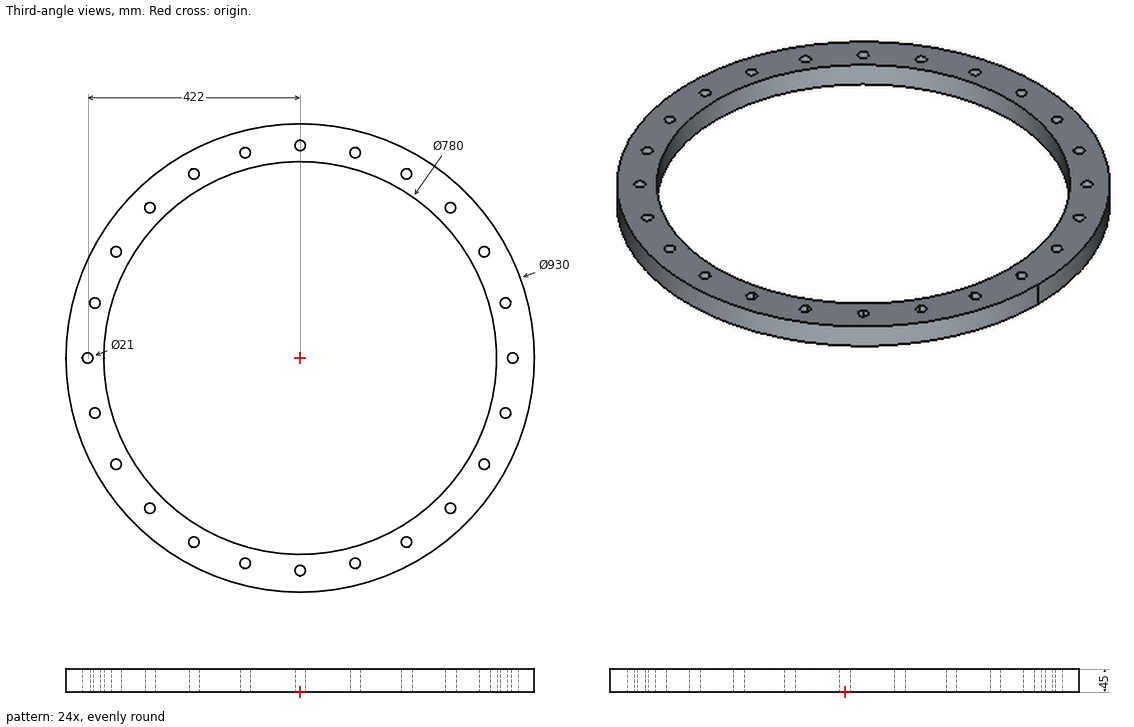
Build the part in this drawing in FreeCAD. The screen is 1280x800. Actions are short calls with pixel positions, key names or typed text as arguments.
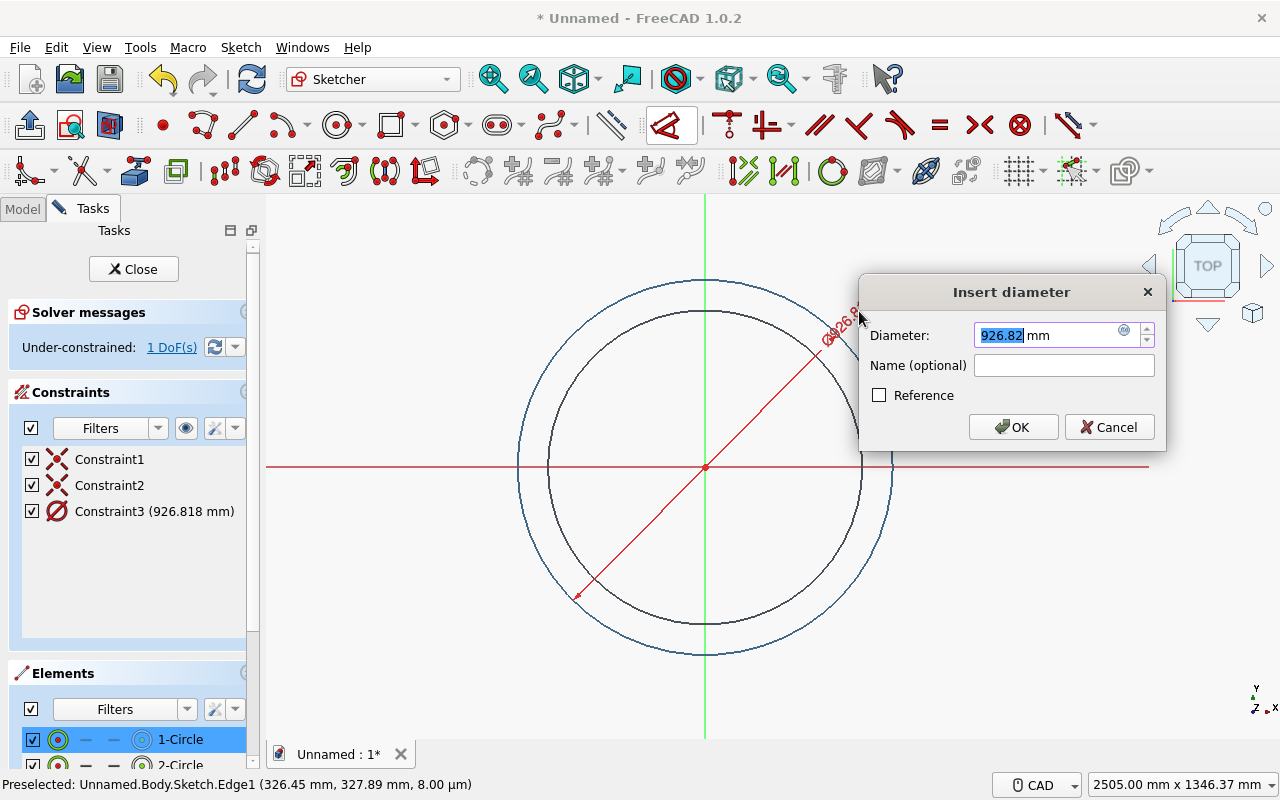
text(930)
key(Return)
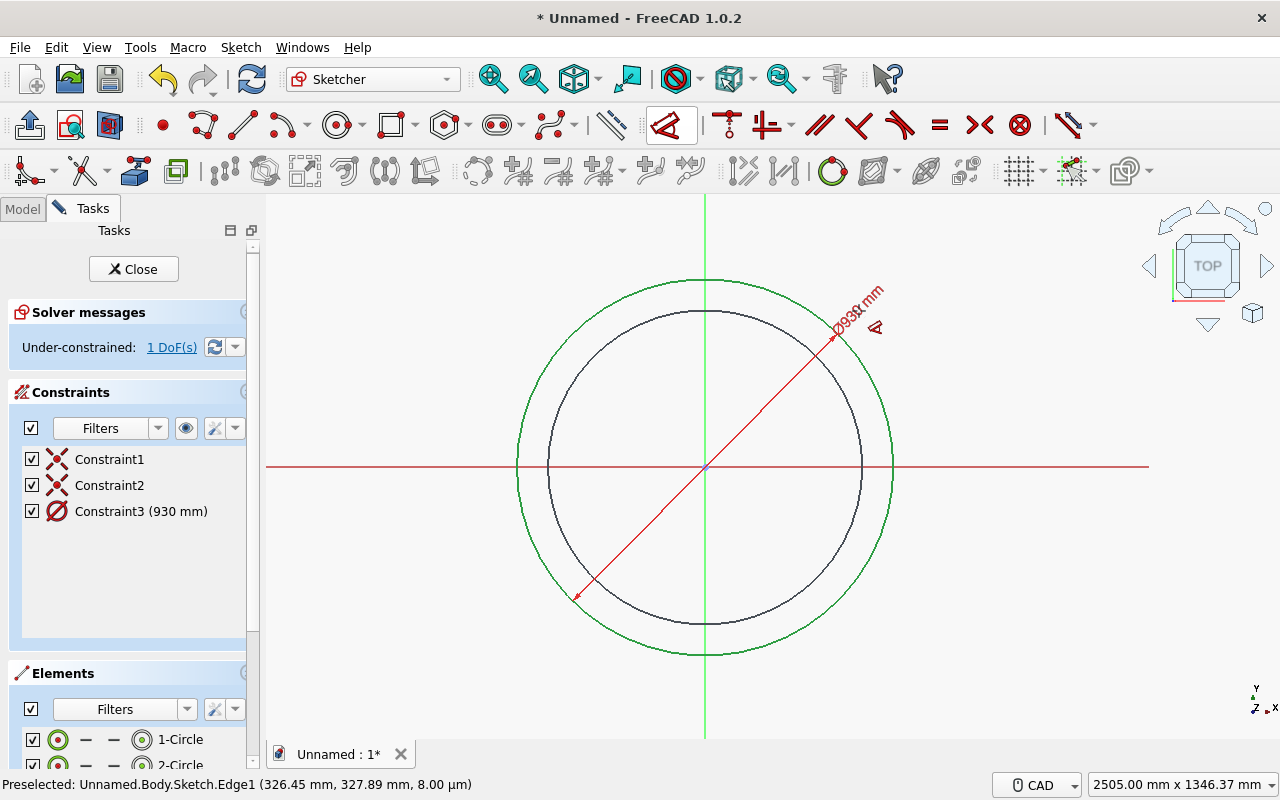
click(816, 356)
click(909, 407)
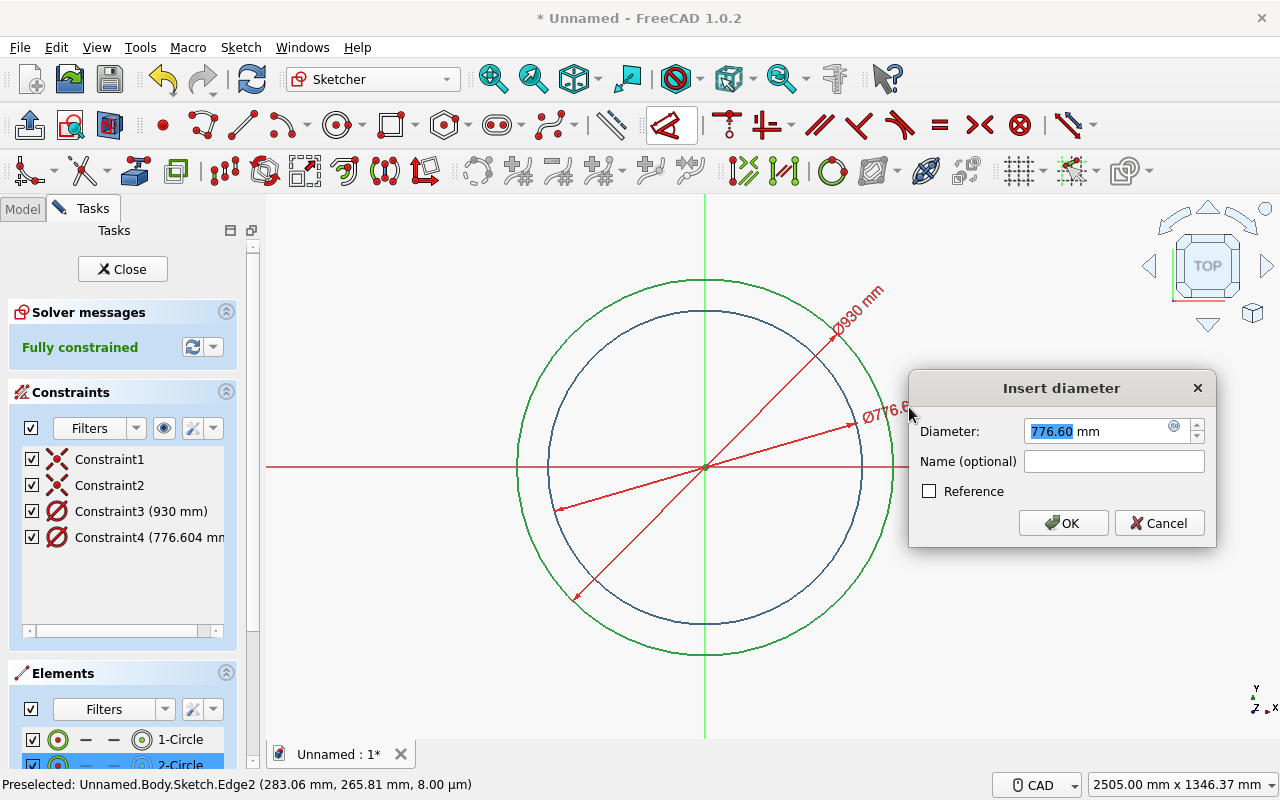
text(780)
key(Return)
key(Escape)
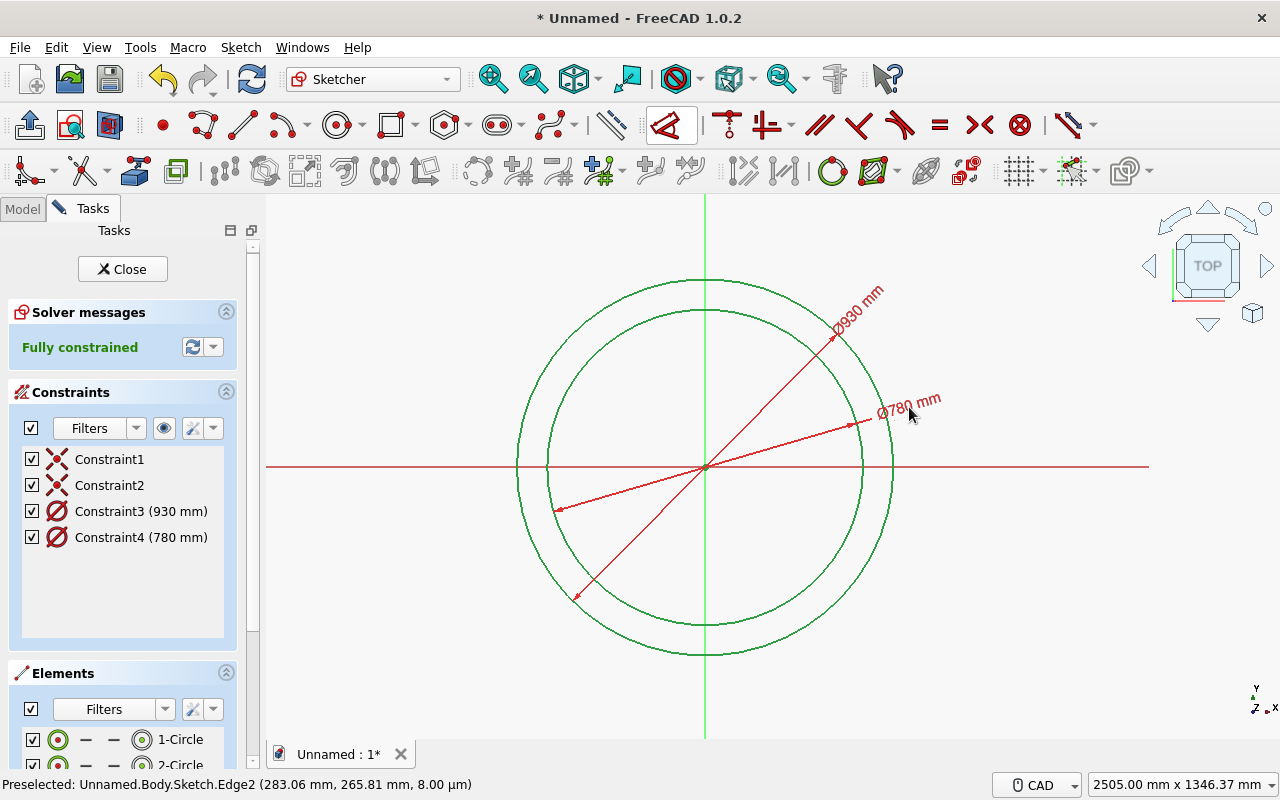
click(123, 269)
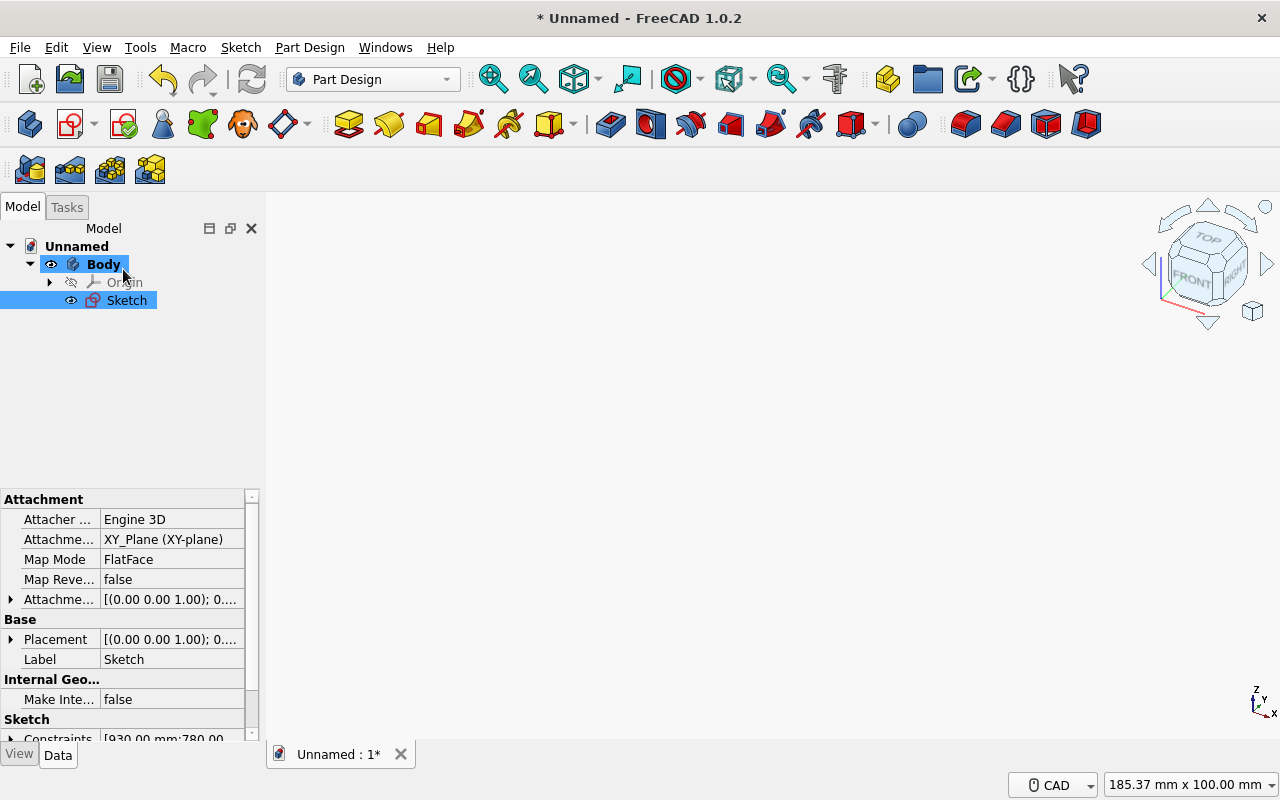
click(350, 124)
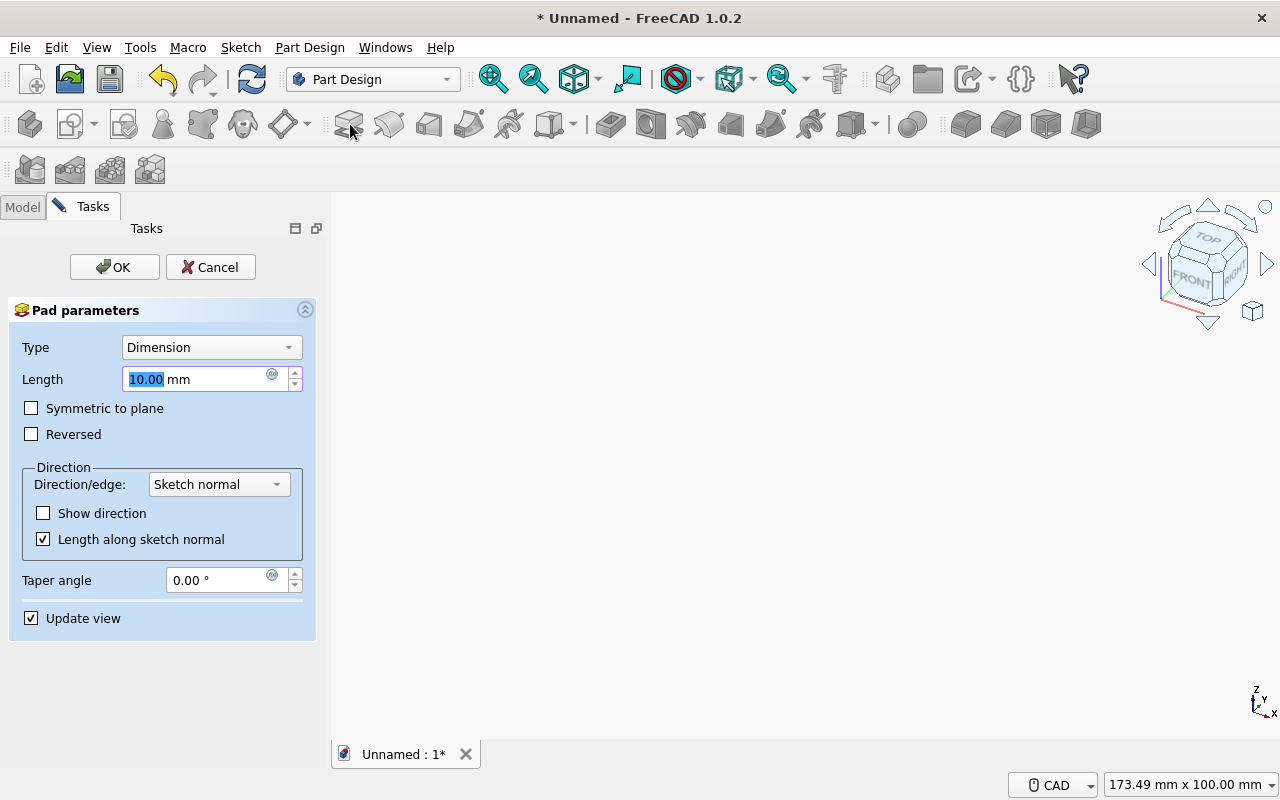
text(45)
key(Tab)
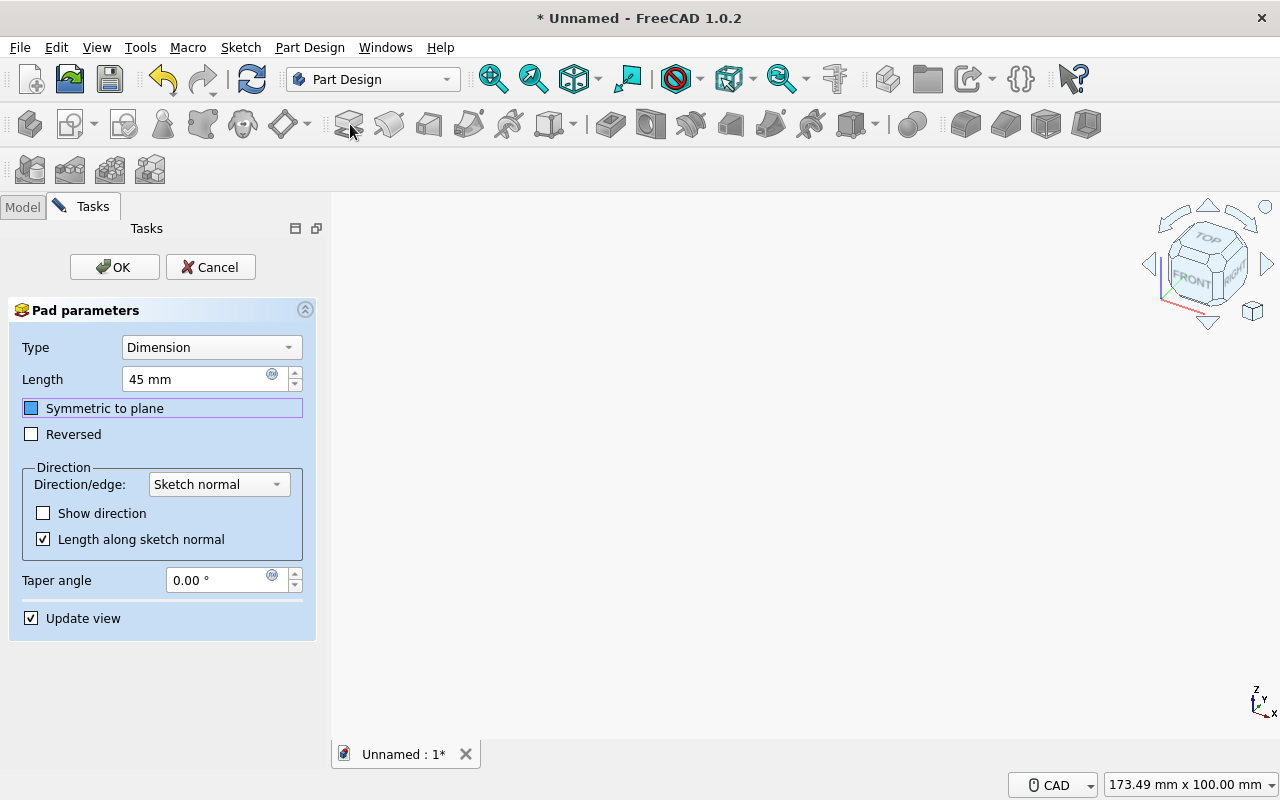
click(115, 267)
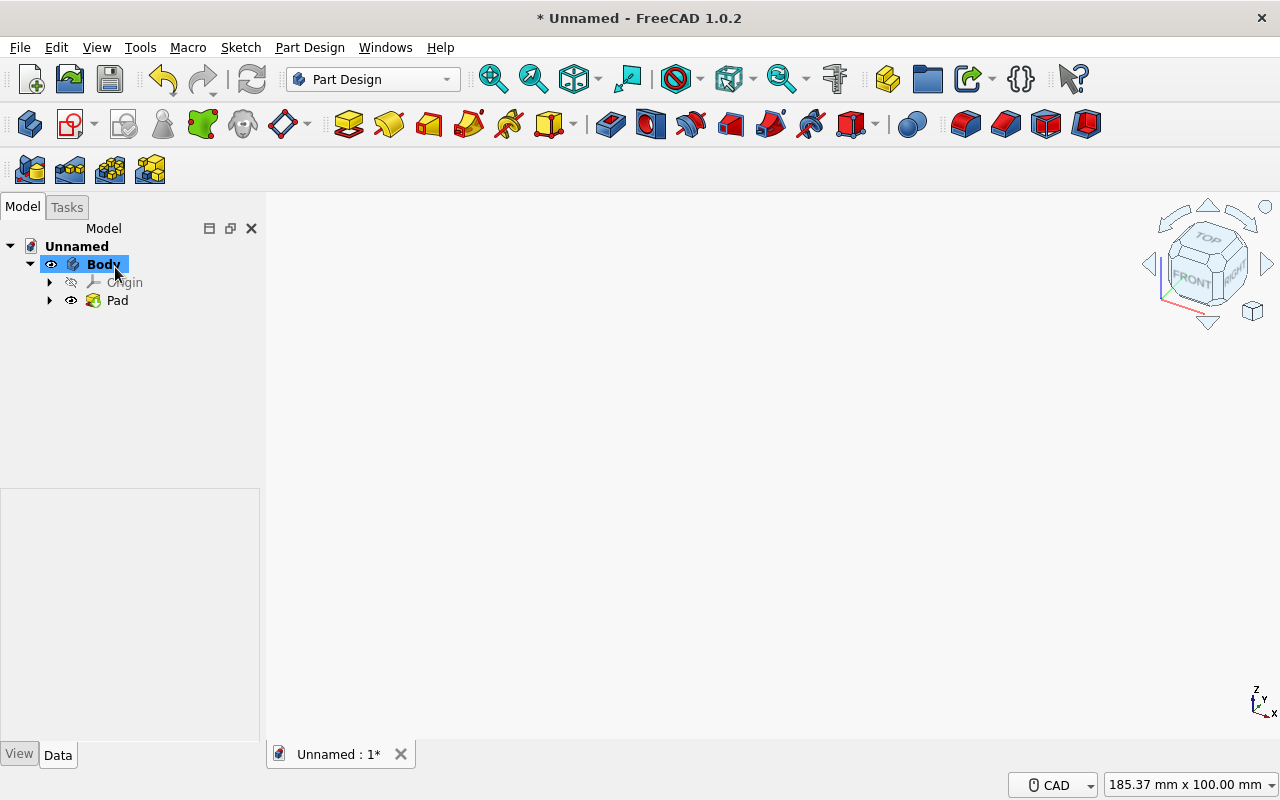
click(494, 80)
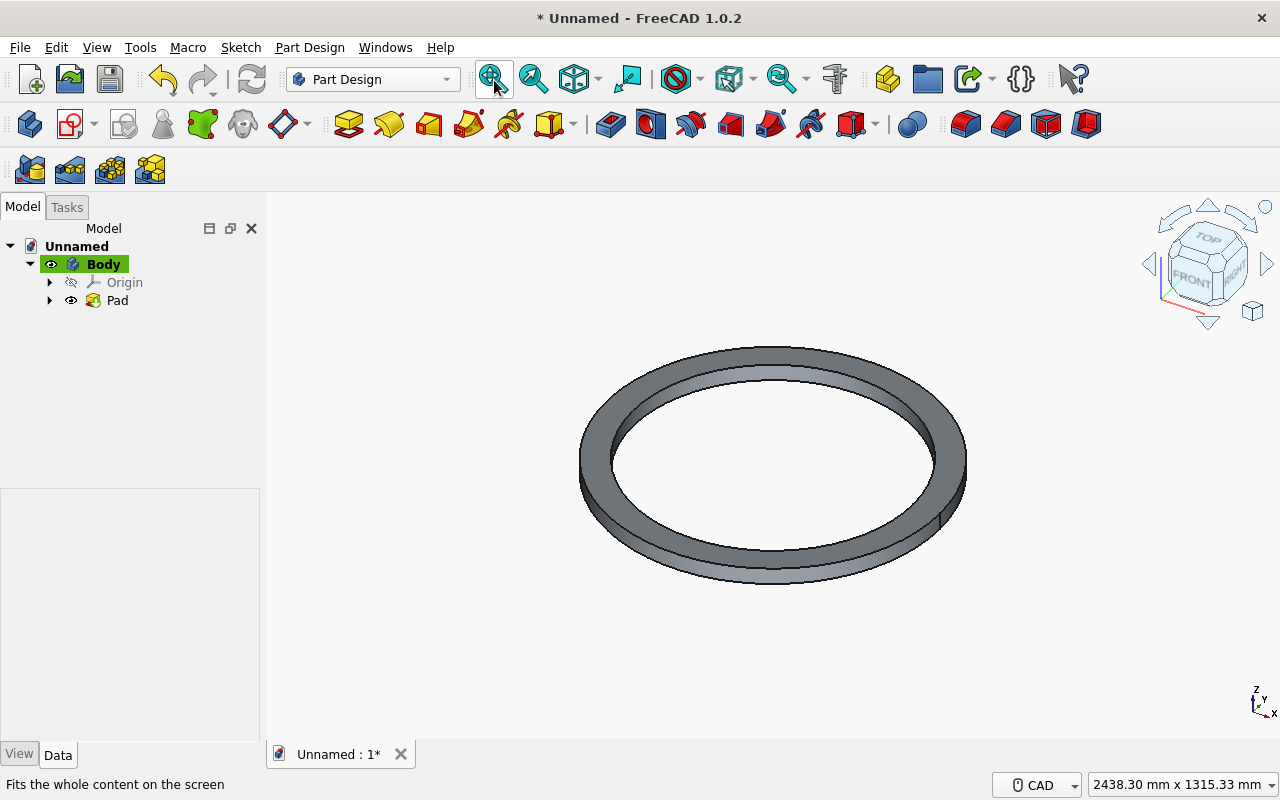
click(944, 477)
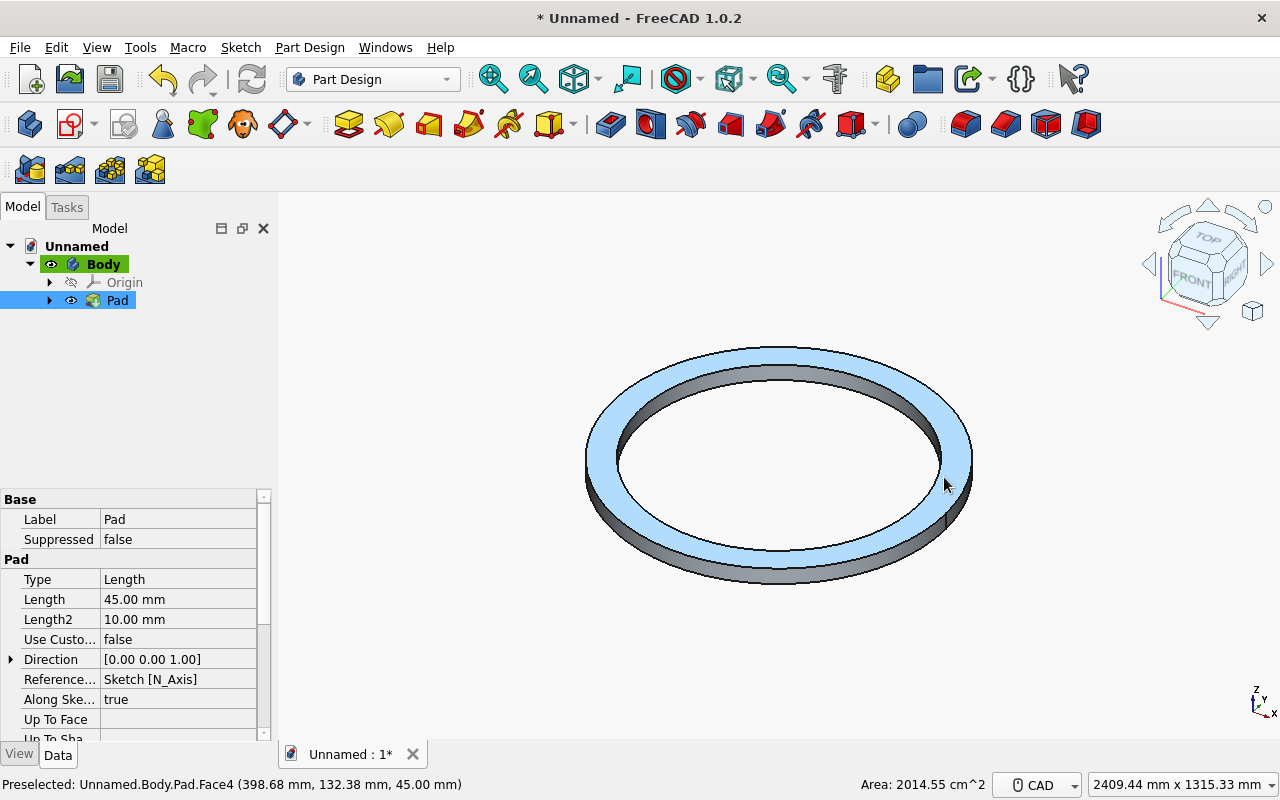
click(70, 124)